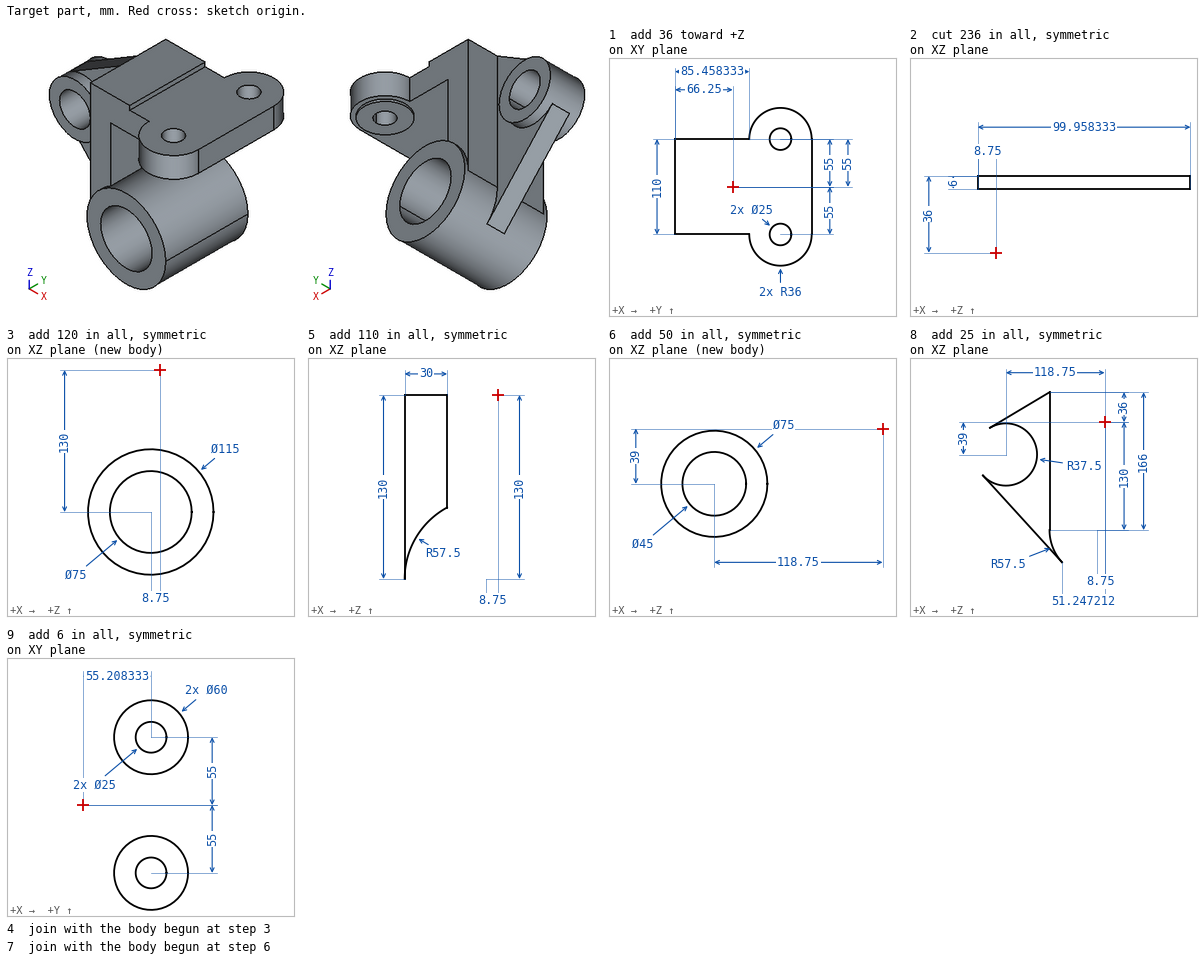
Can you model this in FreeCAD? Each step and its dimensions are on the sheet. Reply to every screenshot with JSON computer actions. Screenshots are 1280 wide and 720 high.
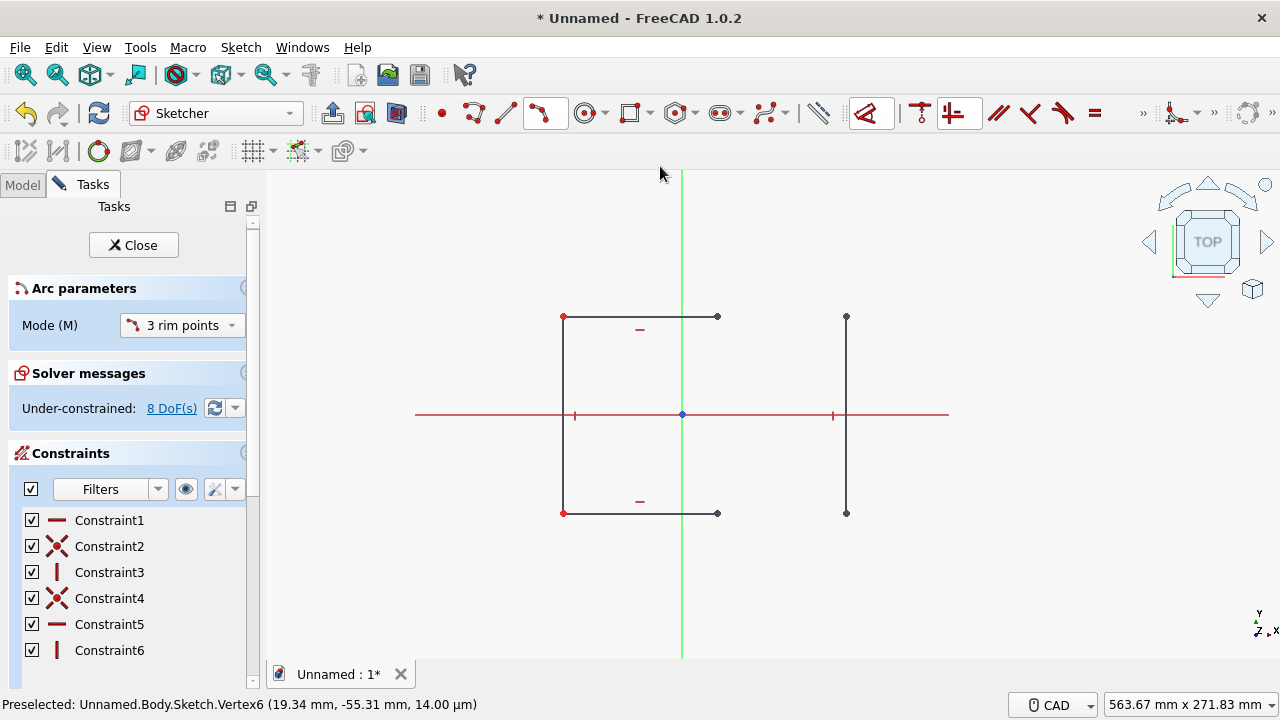
{"action": "left_click", "coordinate": [717, 514]}
{"action": "left_click", "coordinate": [846, 514]}
{"action": "left_click", "coordinate": [782, 578]}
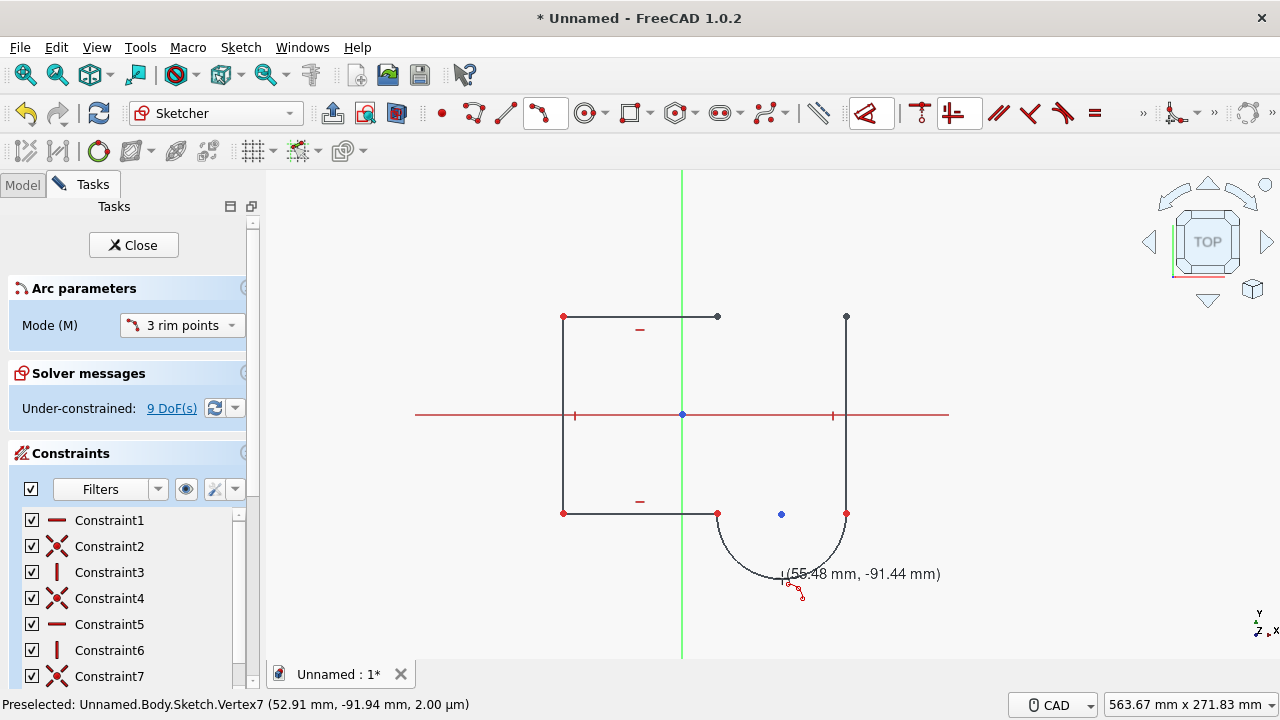
{"action": "left_click", "coordinate": [846, 317]}
{"action": "left_click", "coordinate": [717, 317]}
{"action": "left_click", "coordinate": [782, 251]}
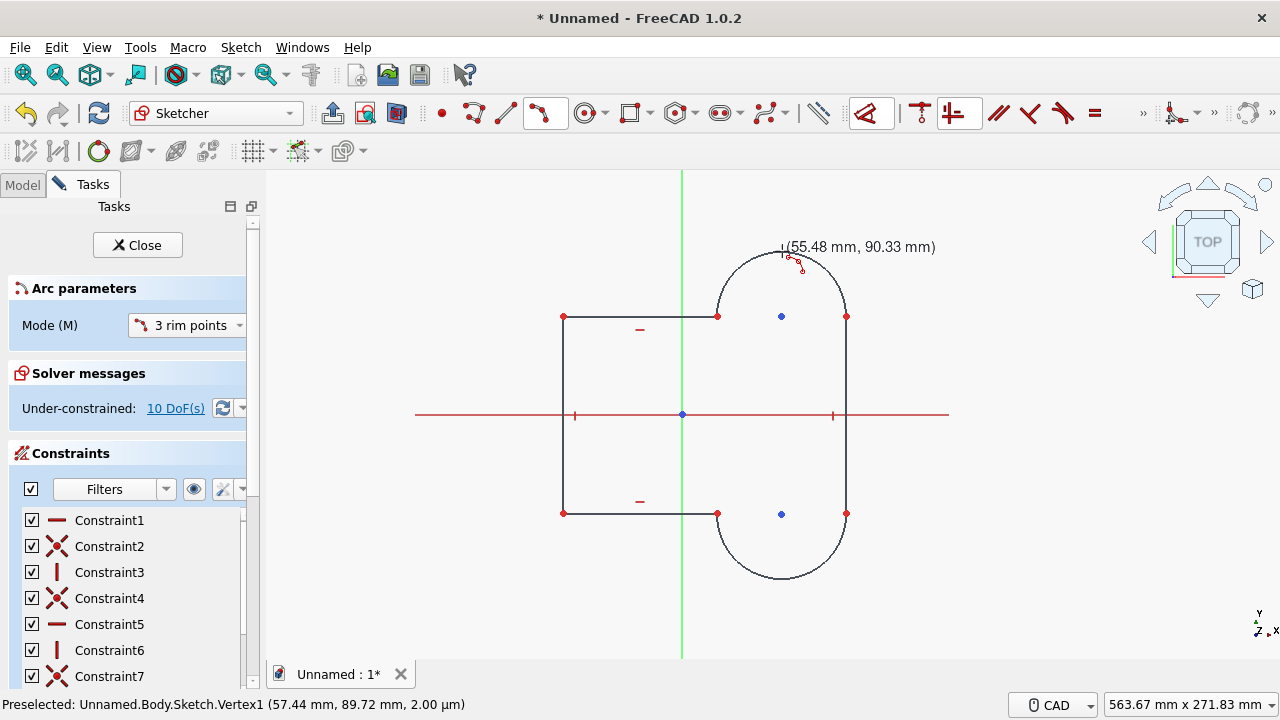
{"action": "left_click", "coordinate": [586, 114]}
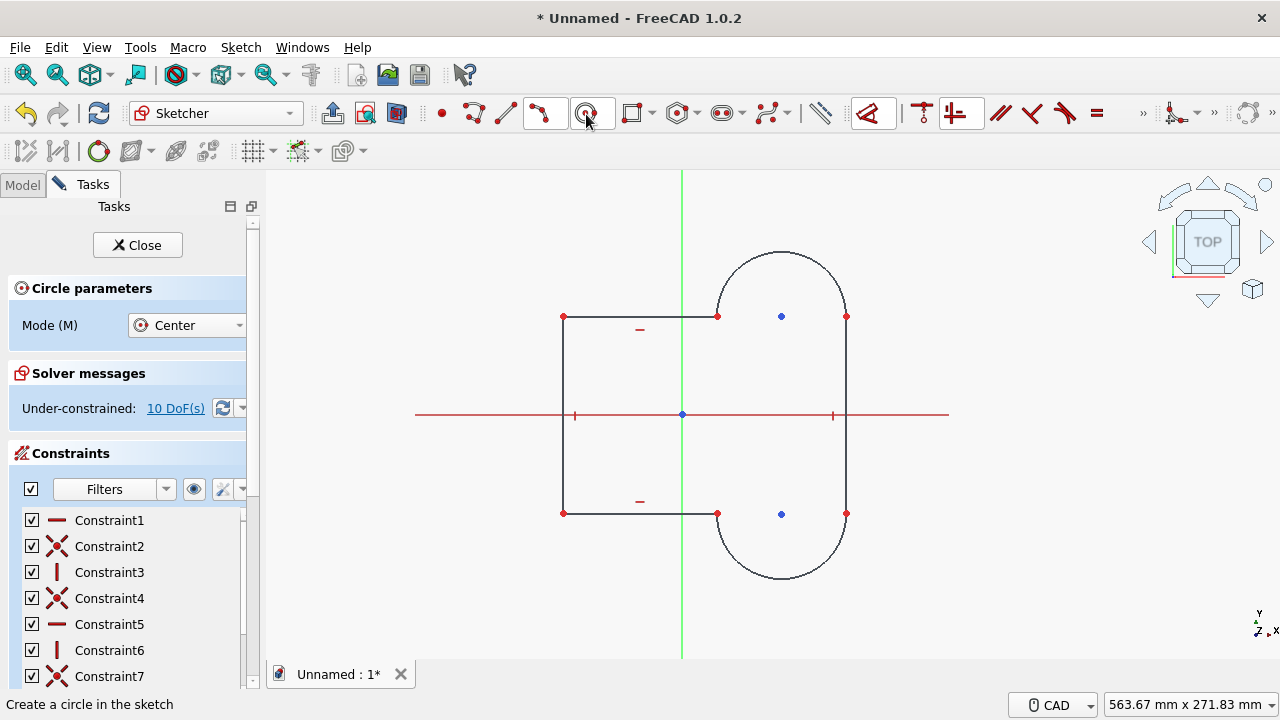
{"action": "left_click", "coordinate": [782, 513]}
{"action": "left_click", "coordinate": [797, 498]}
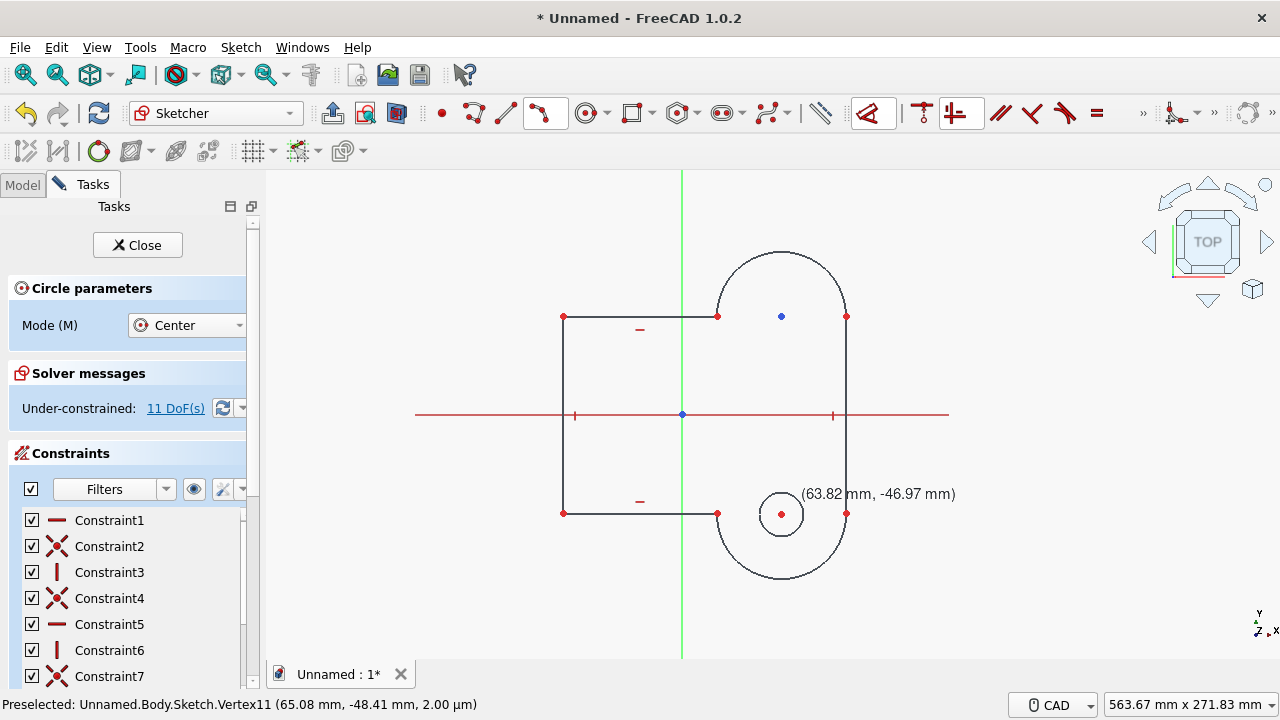
{"action": "left_click", "coordinate": [782, 316]}
{"action": "left_click", "coordinate": [797, 300]}
{"action": "key", "text": "Escape"}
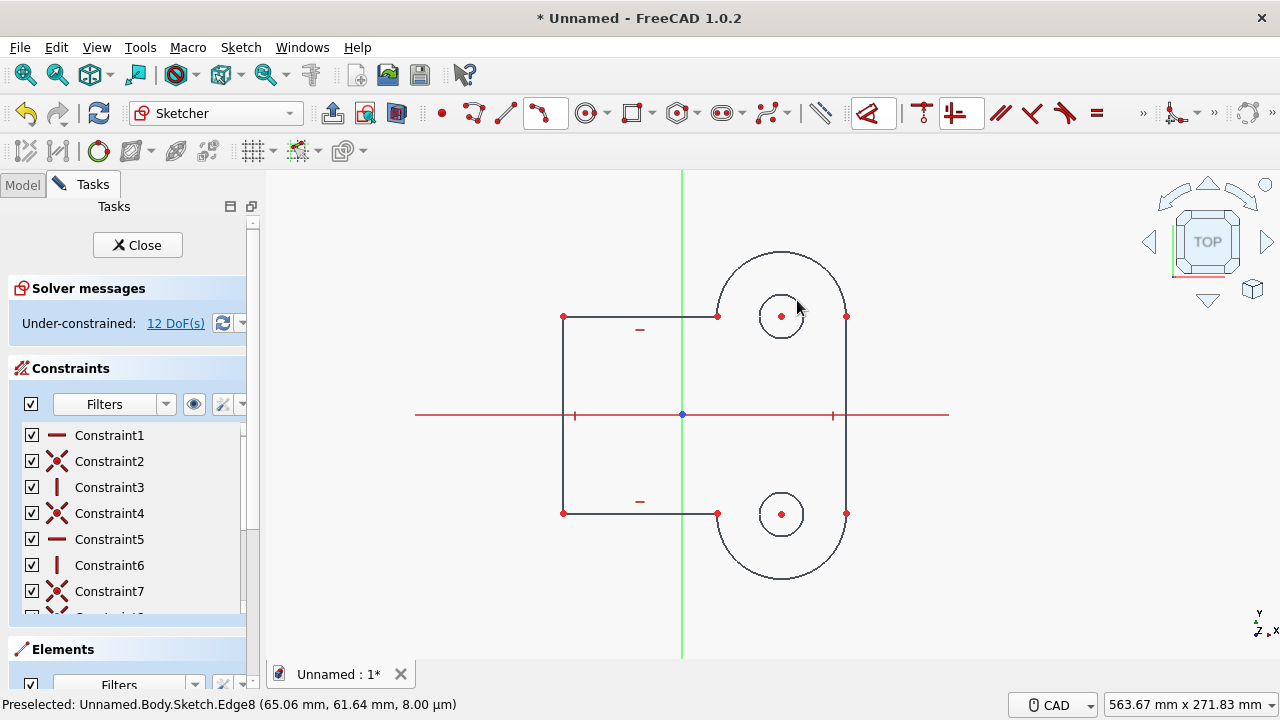
{"action": "left_click", "coordinate": [846, 455]}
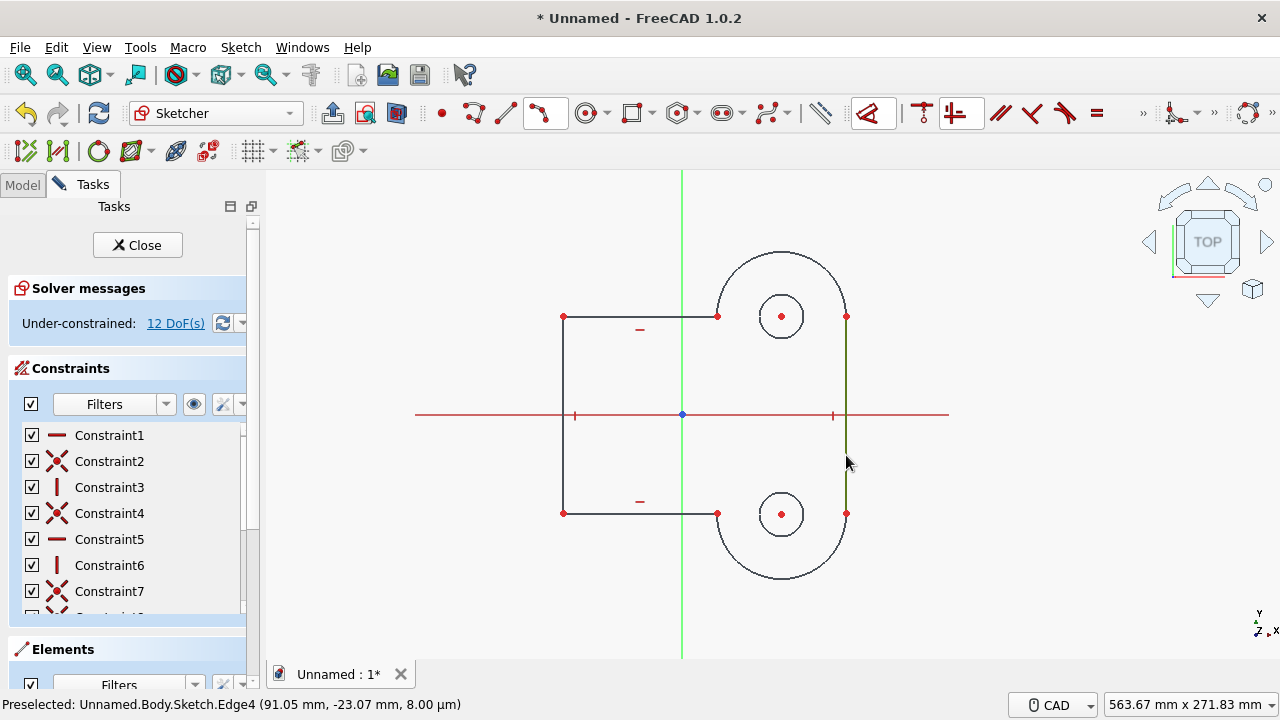
{"action": "left_click", "coordinate": [743, 567]}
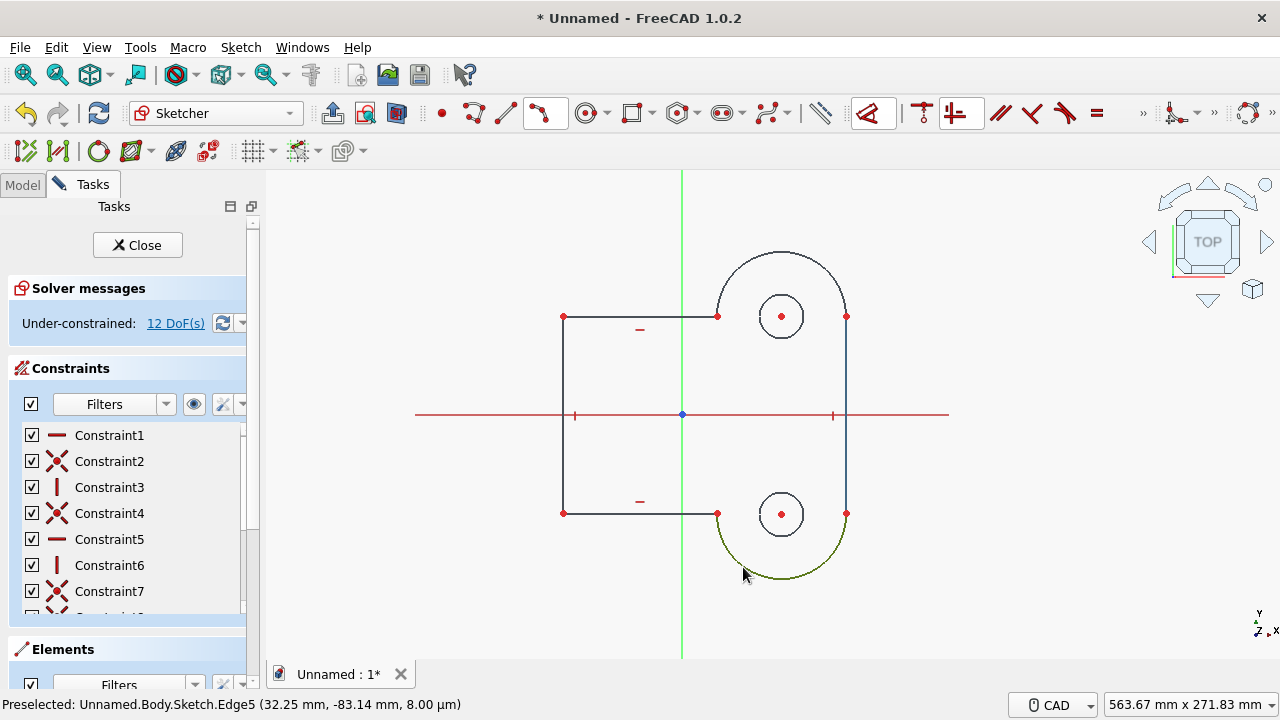
{"action": "key", "text": "t"}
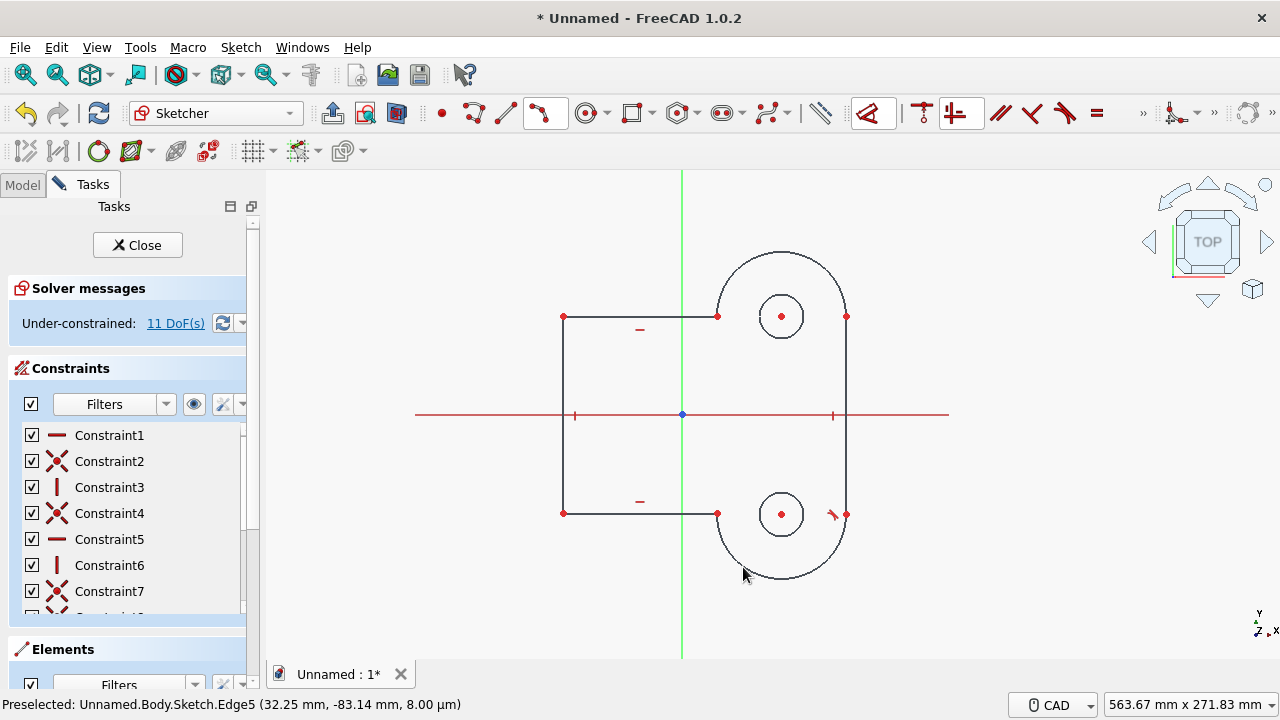
{"action": "left_click", "coordinate": [846, 455]}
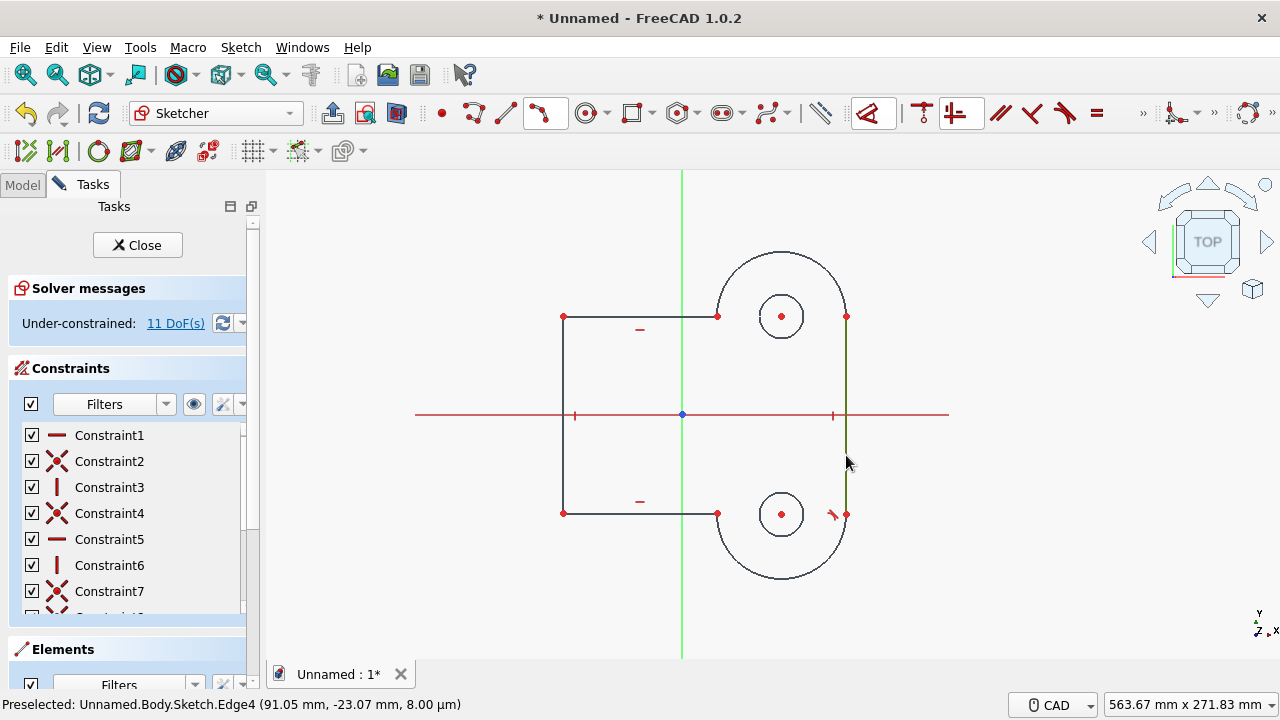
{"action": "left_click", "coordinate": [820, 264]}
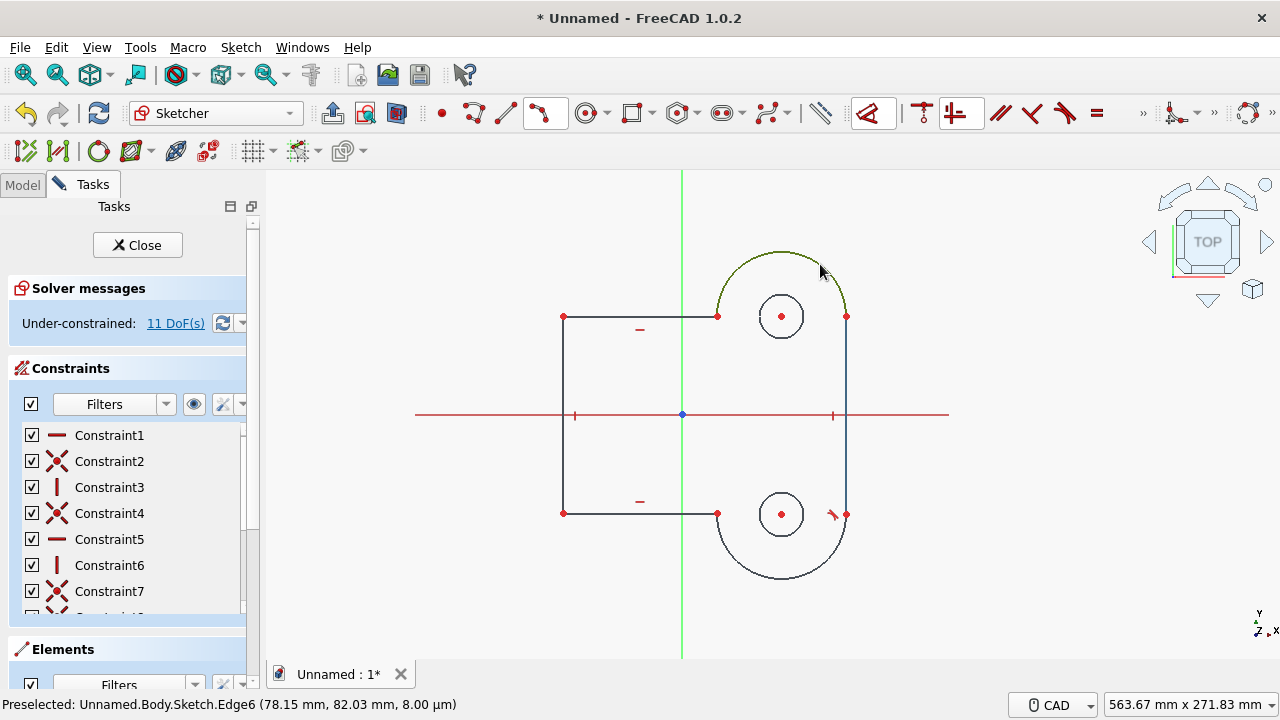
{"action": "left_click", "coordinate": [1066, 114]}